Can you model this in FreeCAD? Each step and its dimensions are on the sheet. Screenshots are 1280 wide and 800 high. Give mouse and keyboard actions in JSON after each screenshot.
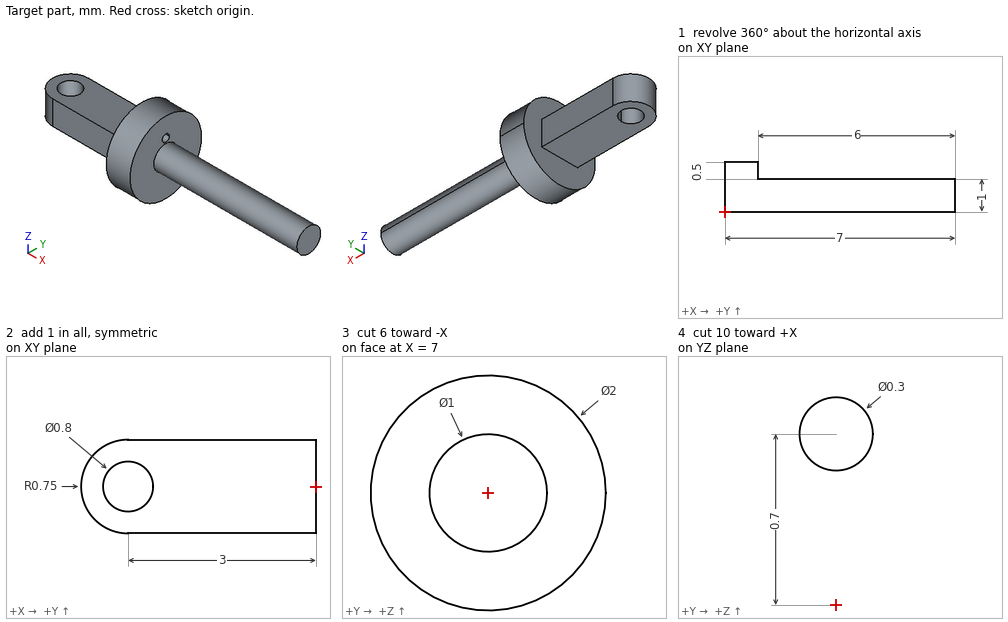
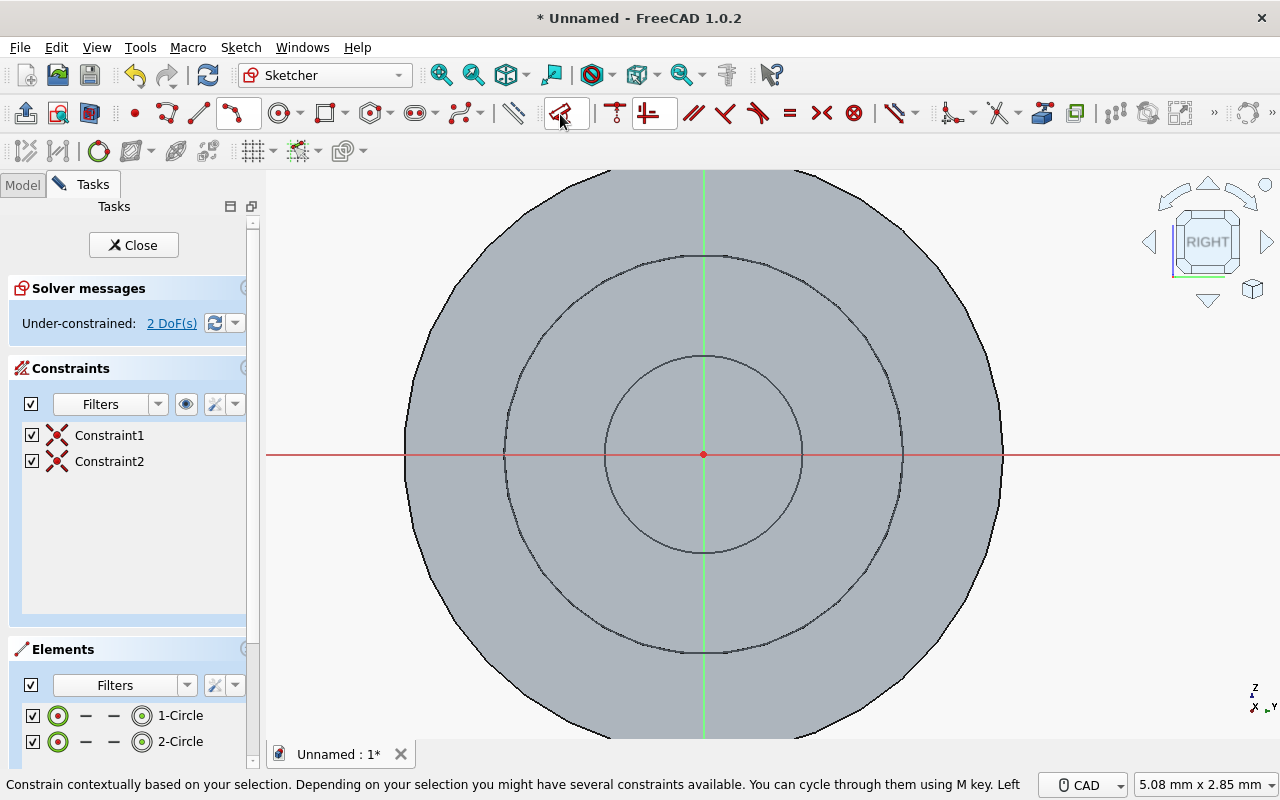
{"action": "left_click", "coordinate": [844, 313]}
{"action": "left_click", "coordinate": [867, 290]}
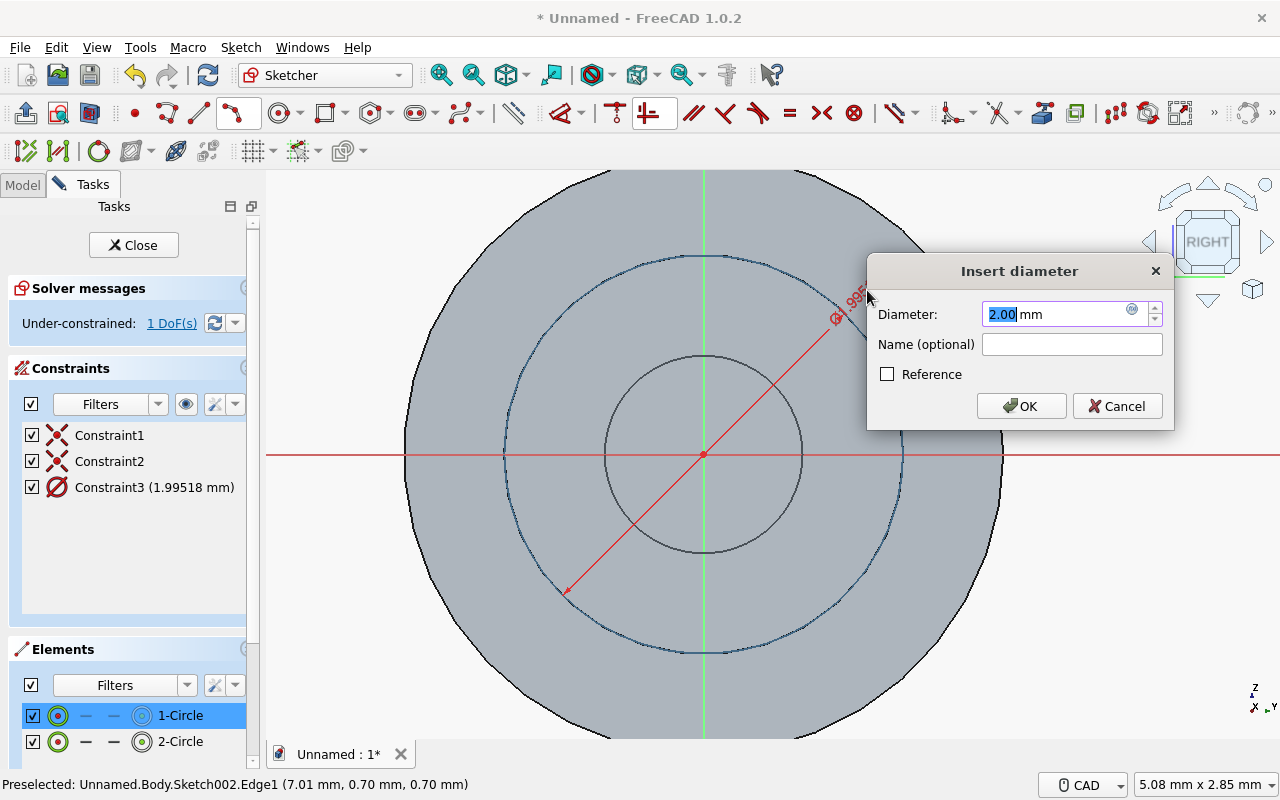
{"action": "type", "text": "2"}
{"action": "key", "text": "Return"}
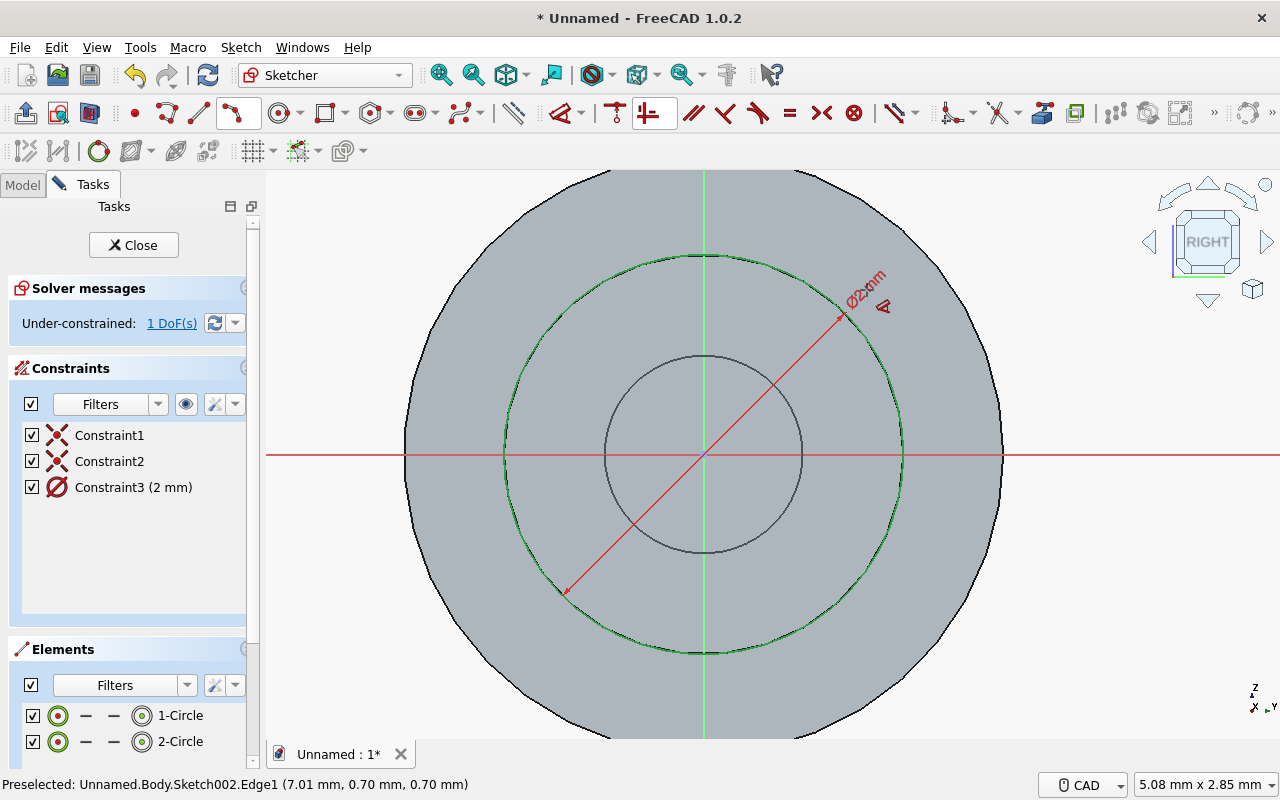
{"action": "left_click", "coordinate": [773, 384]}
{"action": "left_click", "coordinate": [795, 361]}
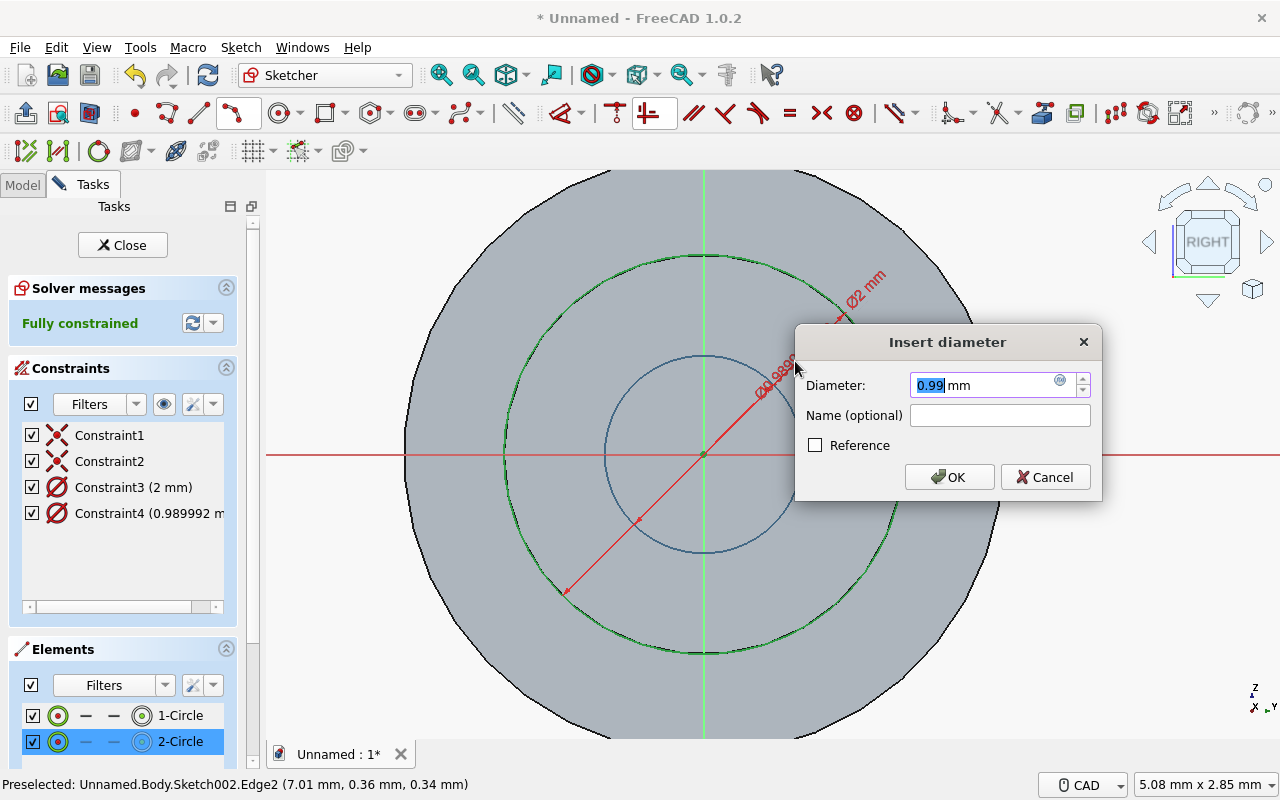
{"action": "type", "text": "1"}
{"action": "key", "text": "Return"}
{"action": "key", "text": "Escape"}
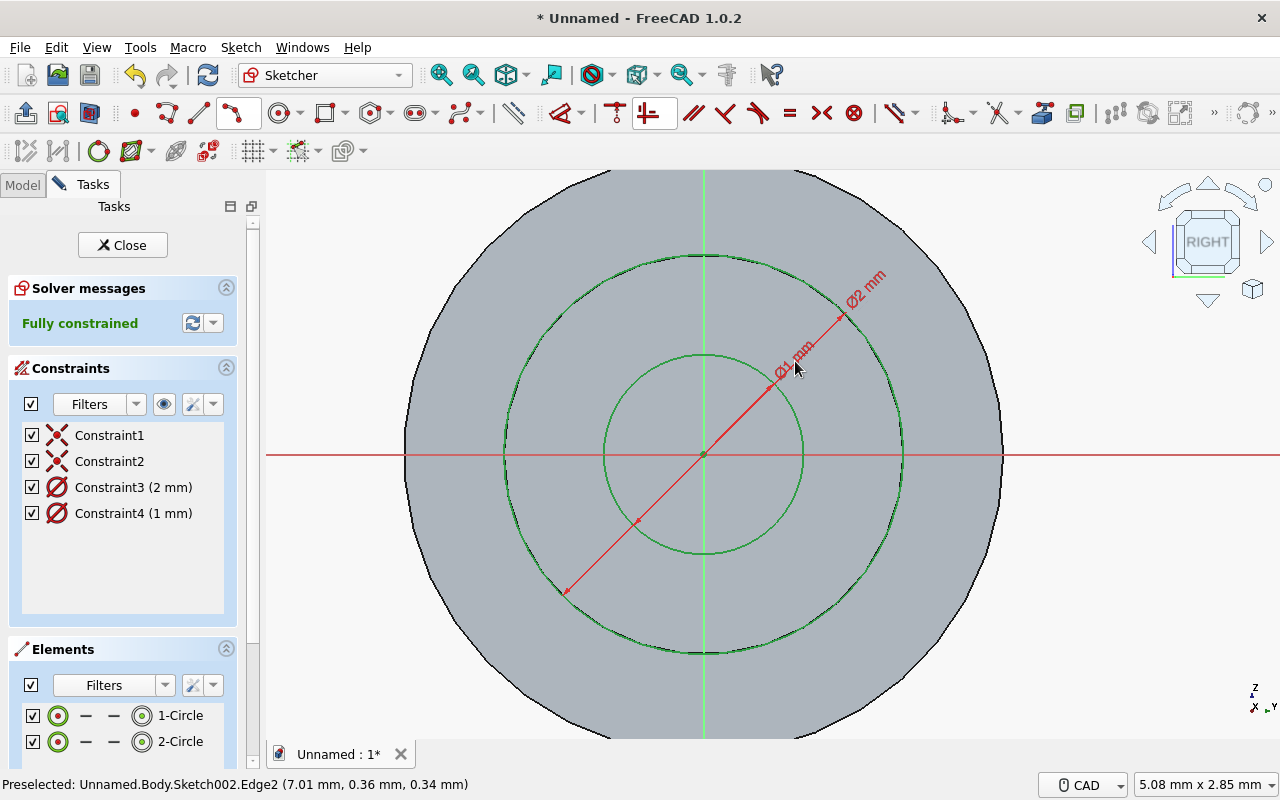
{"action": "left_click", "coordinate": [123, 245]}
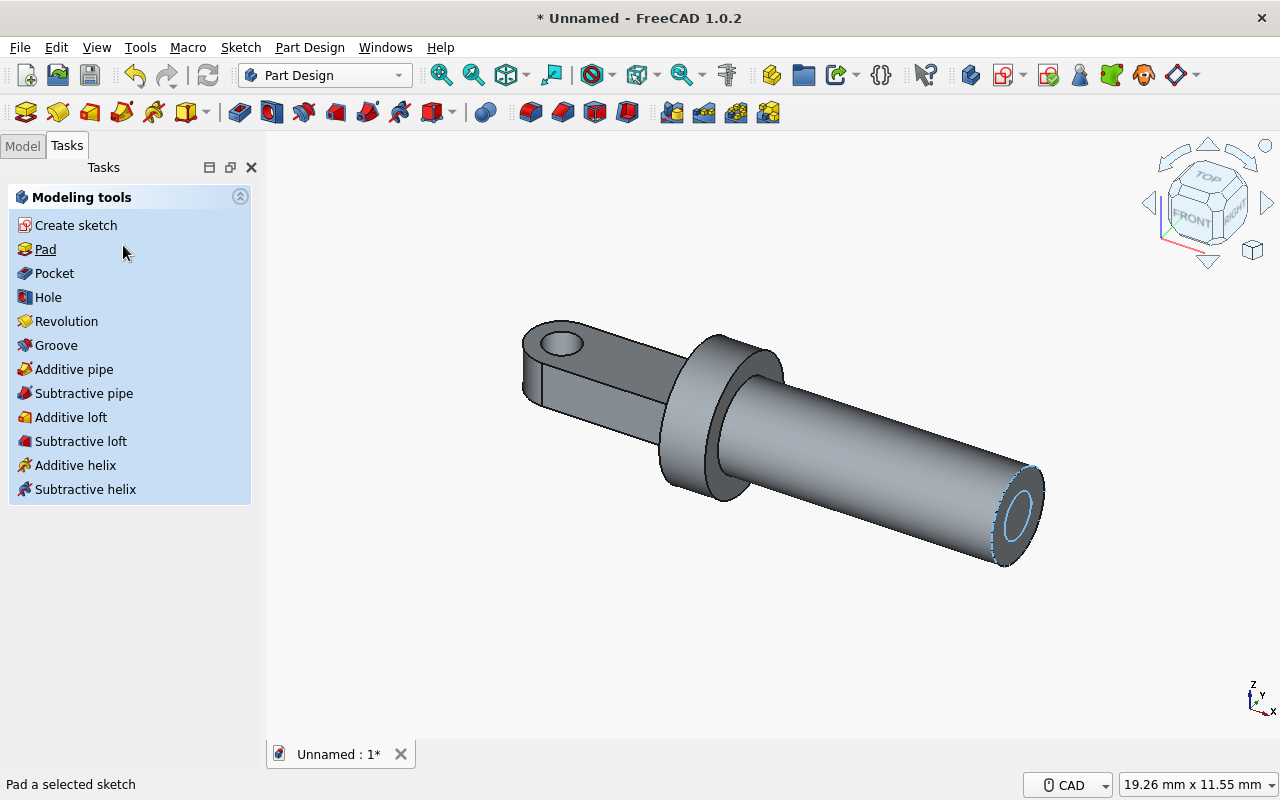
{"action": "left_click", "coordinate": [240, 112]}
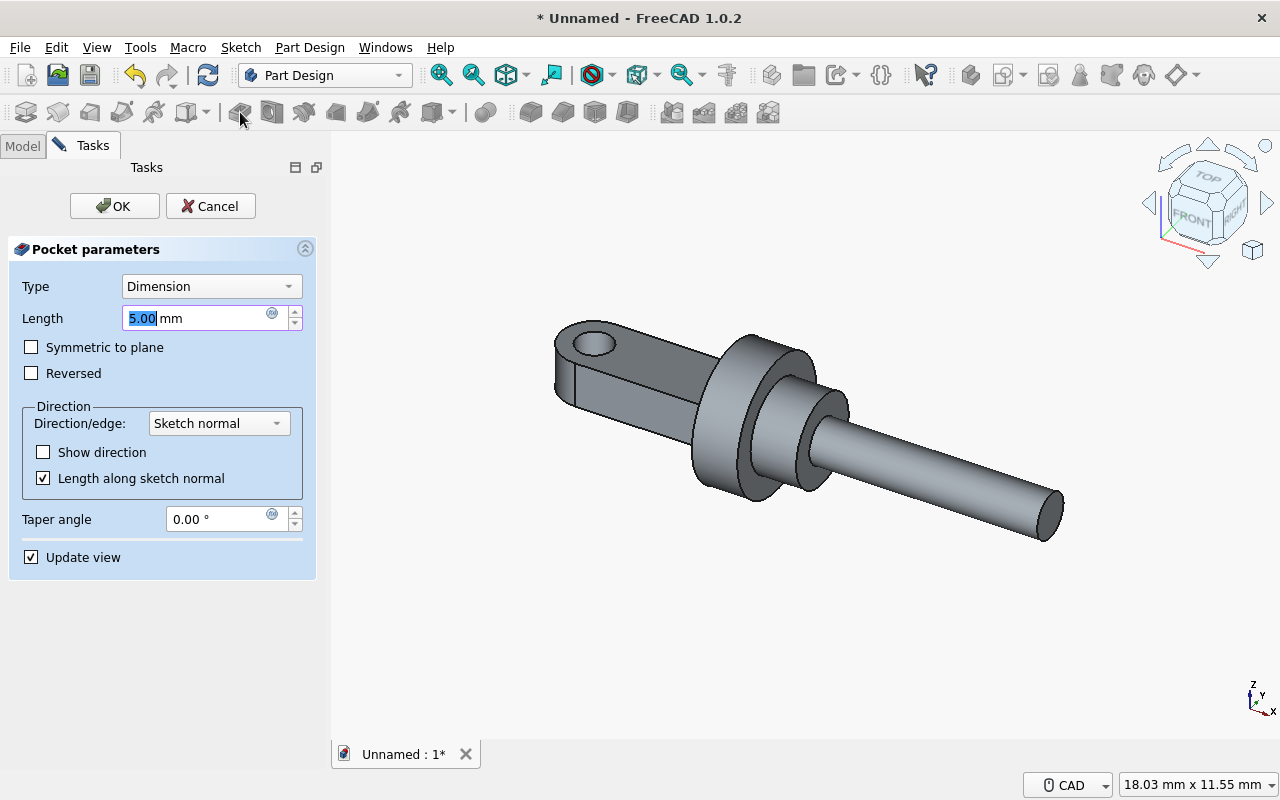
{"action": "type", "text": "6"}
{"action": "key", "text": "Tab"}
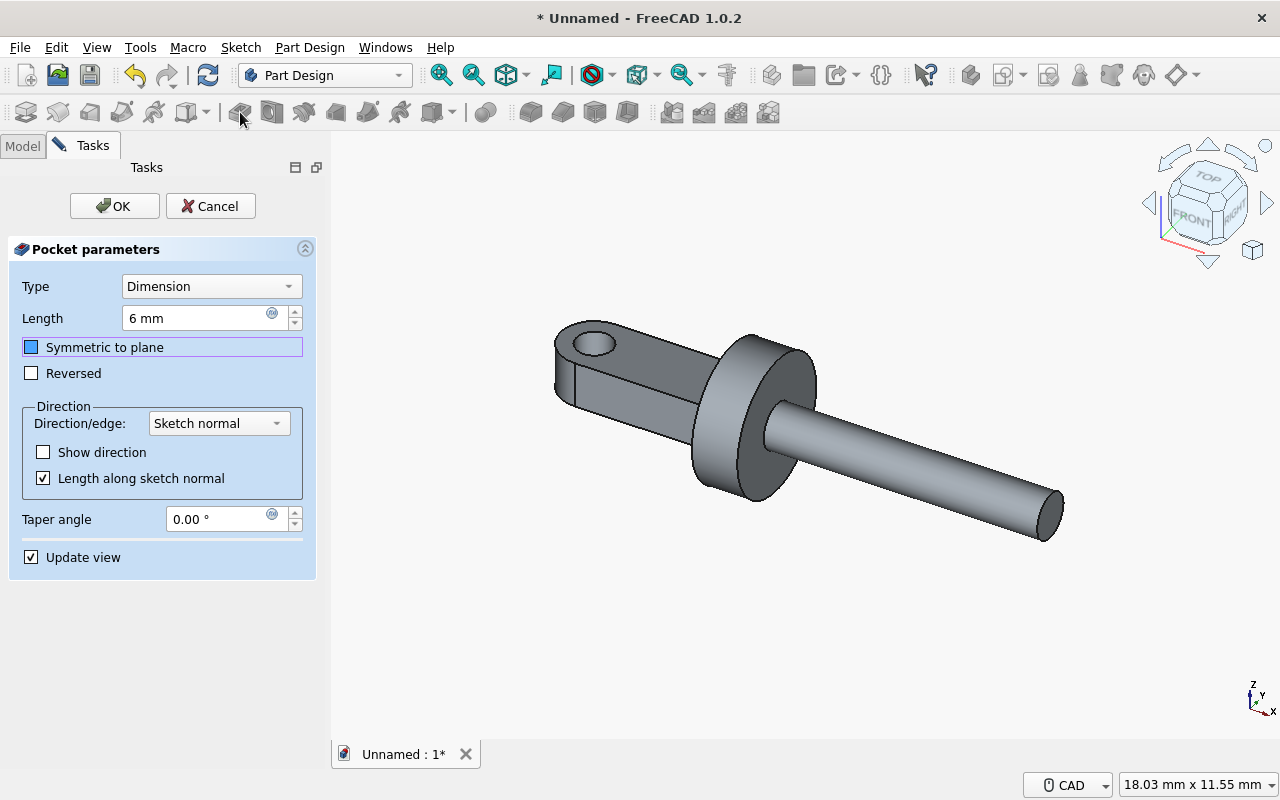
{"action": "left_click", "coordinate": [115, 206]}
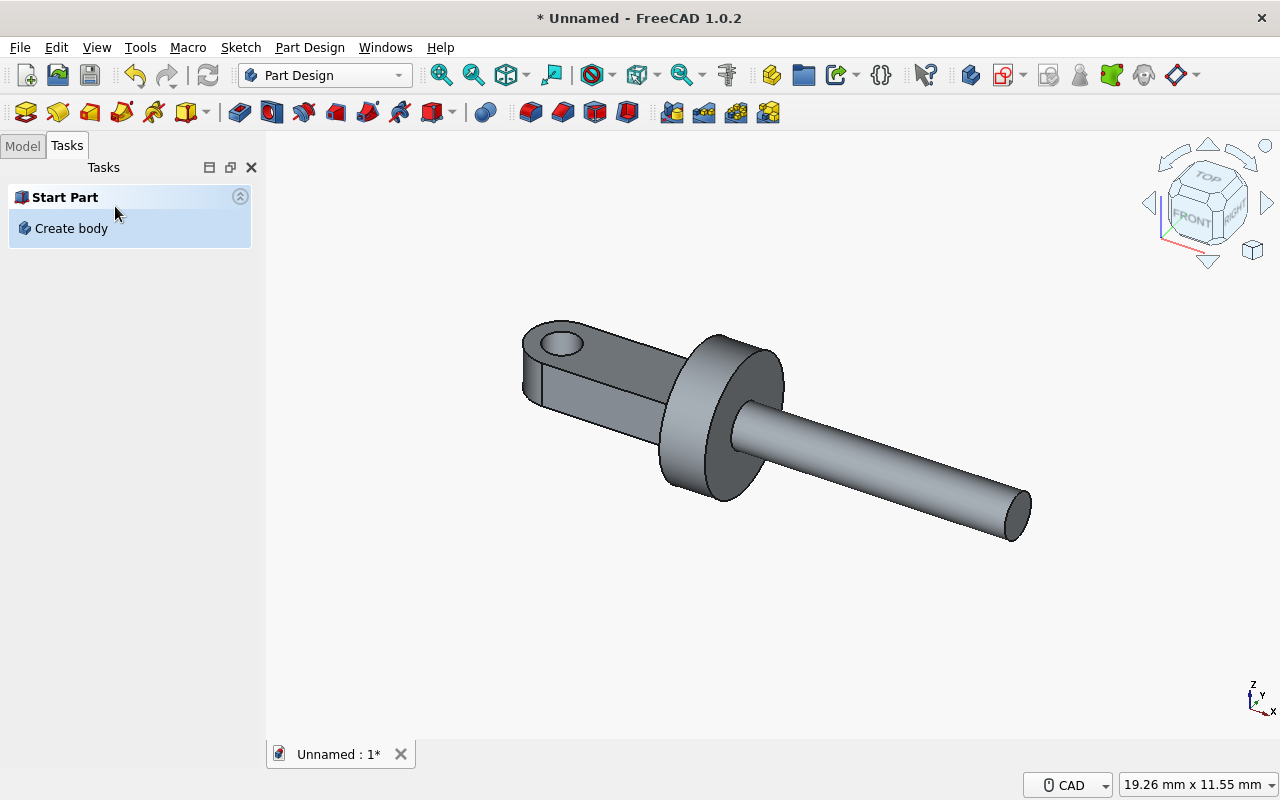
{"action": "left_click", "coordinate": [1004, 76]}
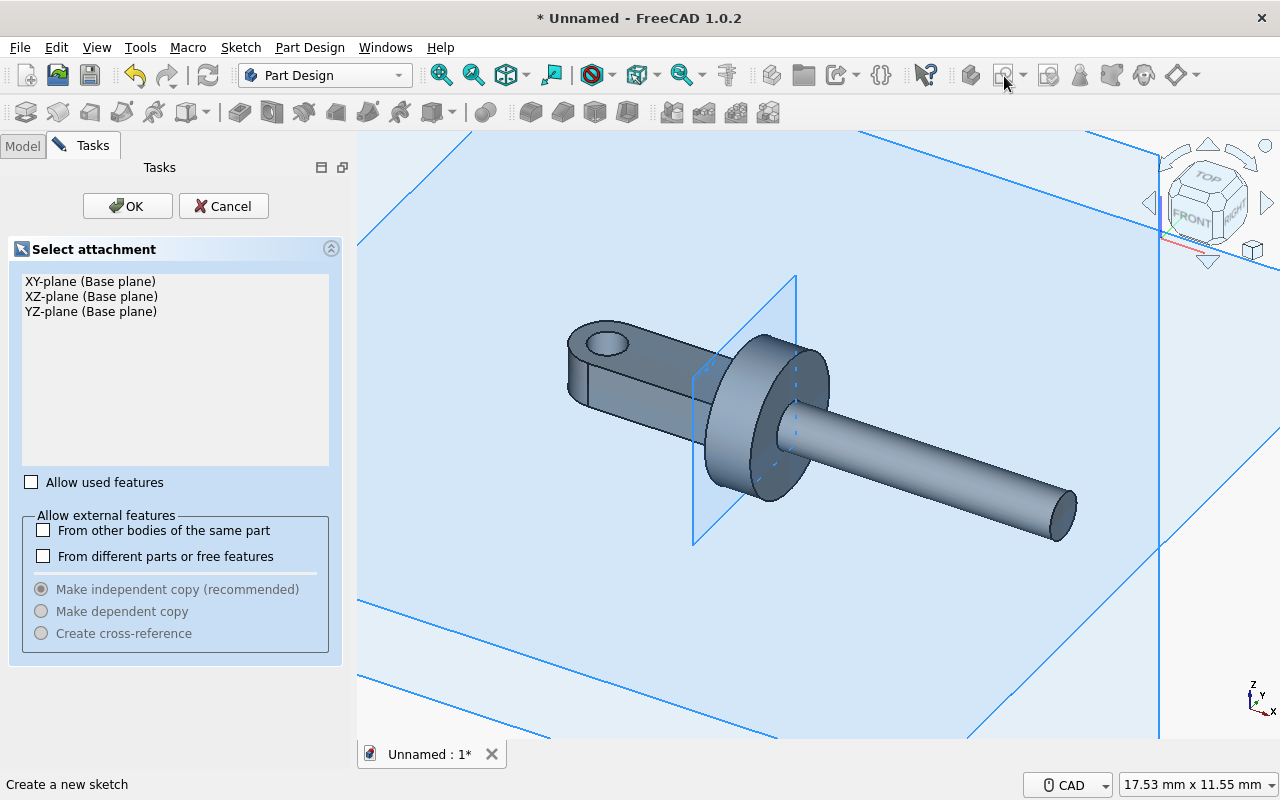
{"action": "left_click", "coordinate": [82, 312]}